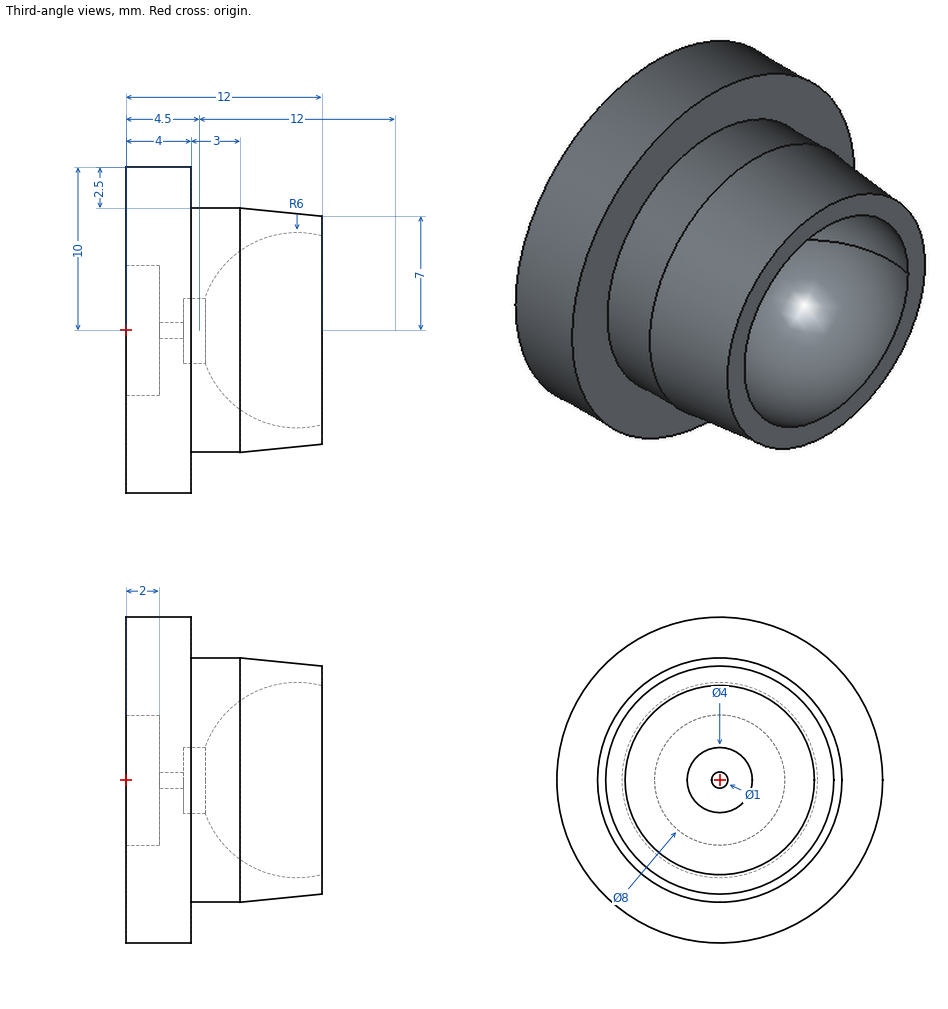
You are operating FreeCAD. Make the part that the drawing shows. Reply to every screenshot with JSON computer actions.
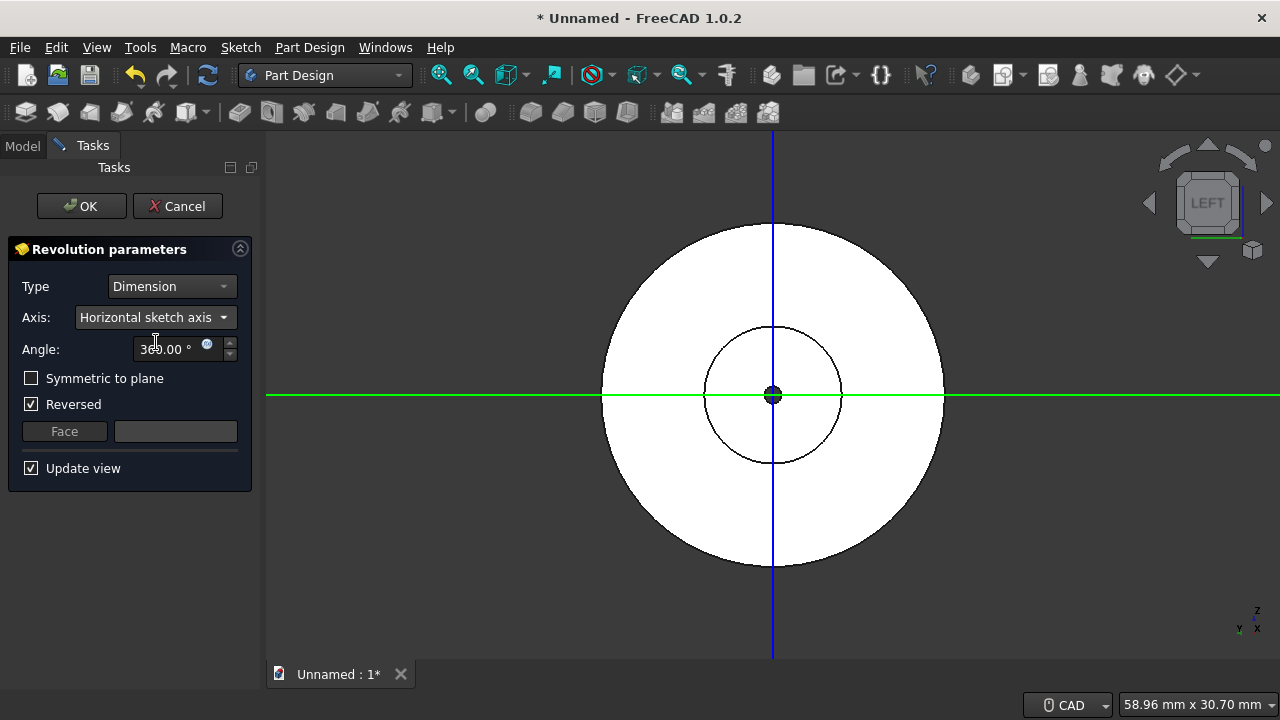
{"action": "left_click", "coordinate": [82, 206]}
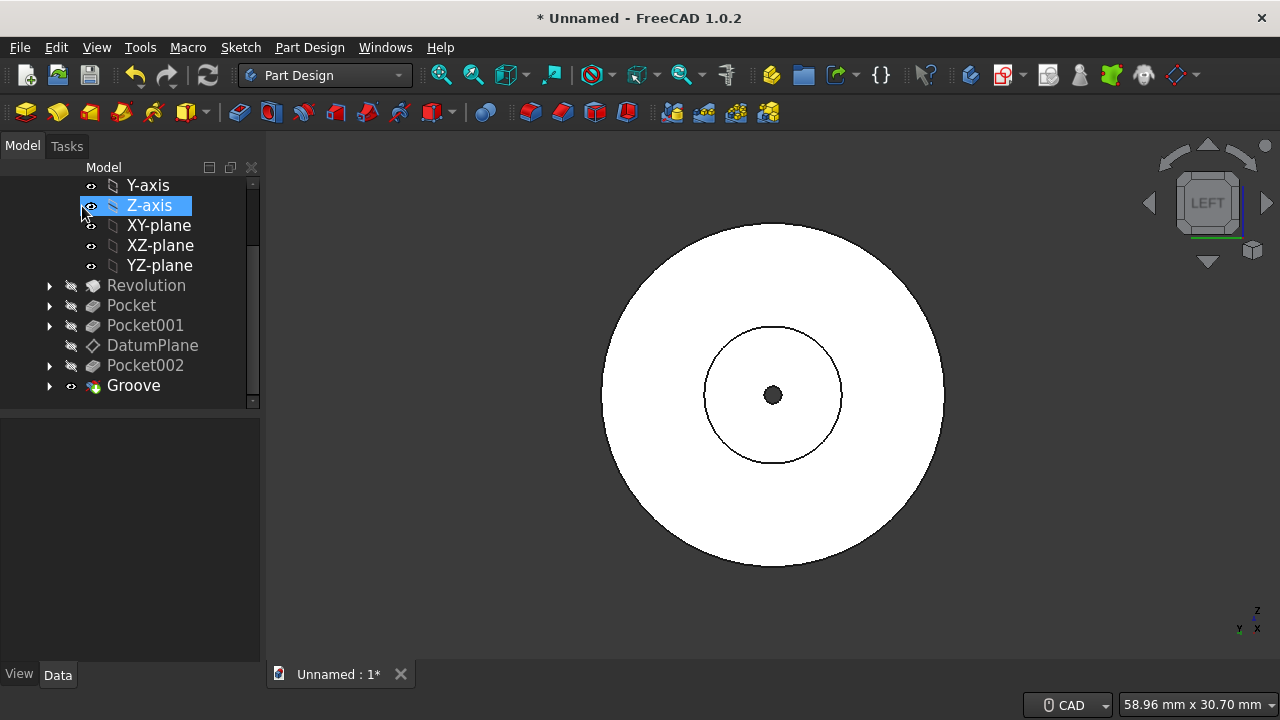
{"action": "key", "text": "0"}